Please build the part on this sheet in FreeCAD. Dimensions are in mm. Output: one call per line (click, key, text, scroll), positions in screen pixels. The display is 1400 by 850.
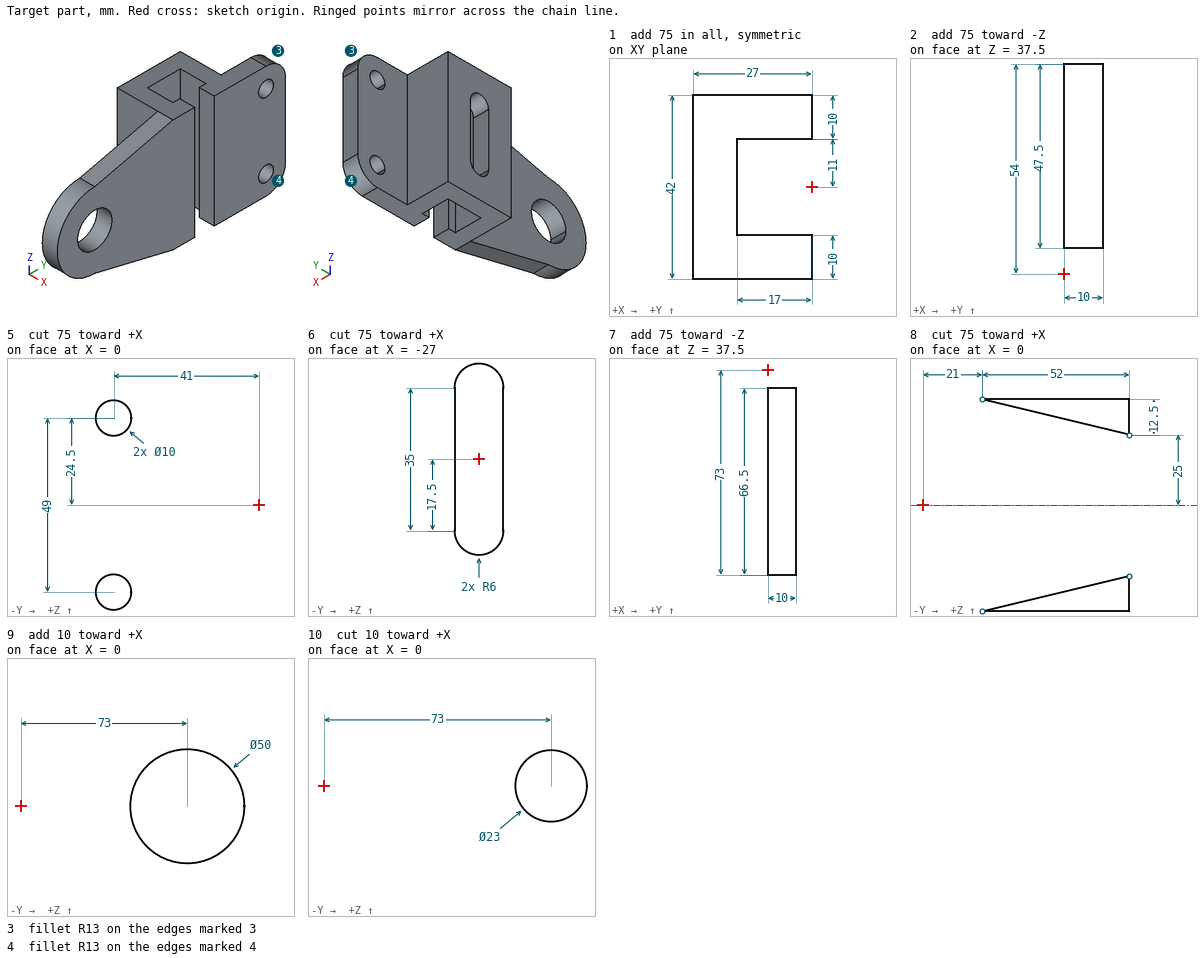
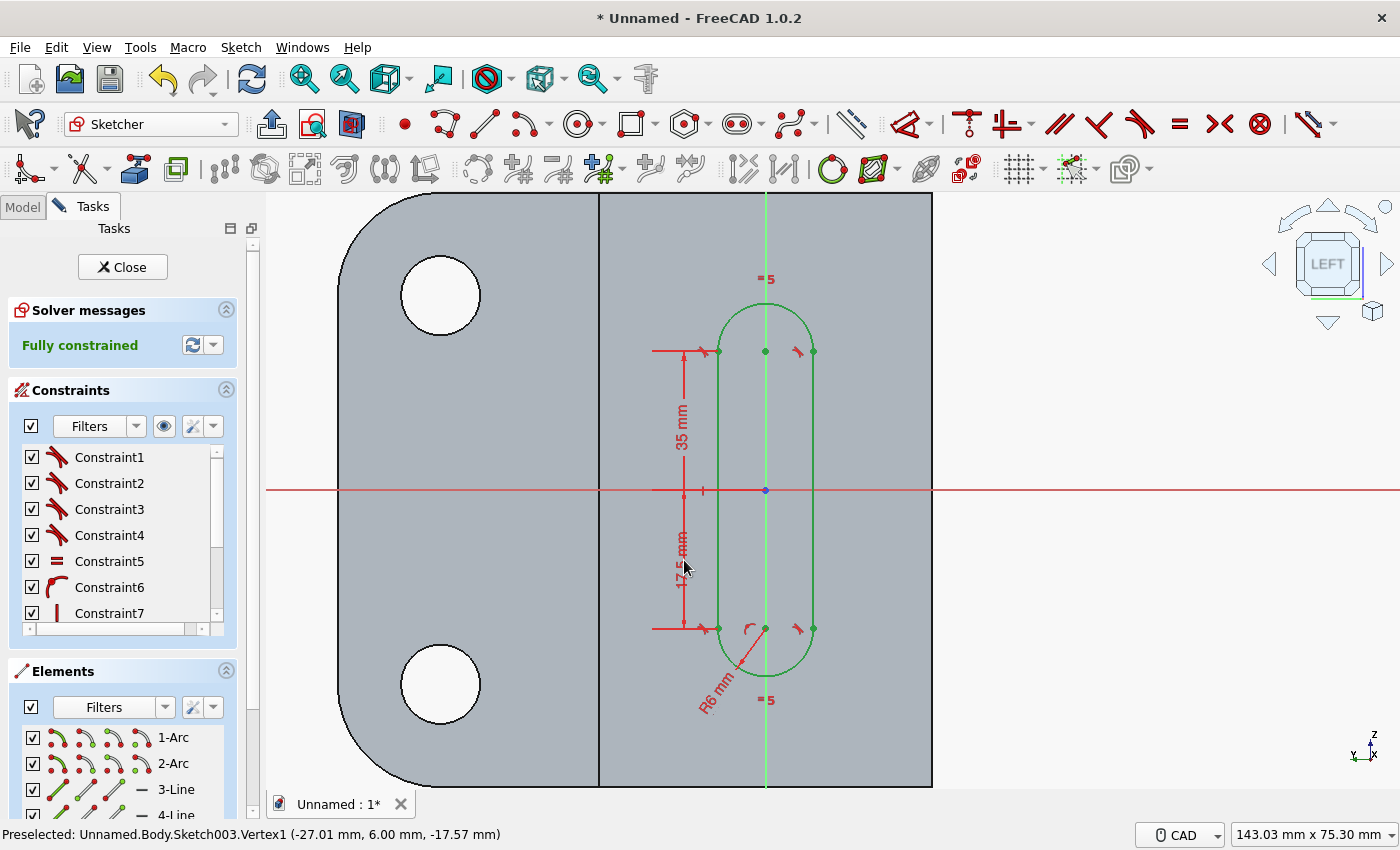
click(123, 267)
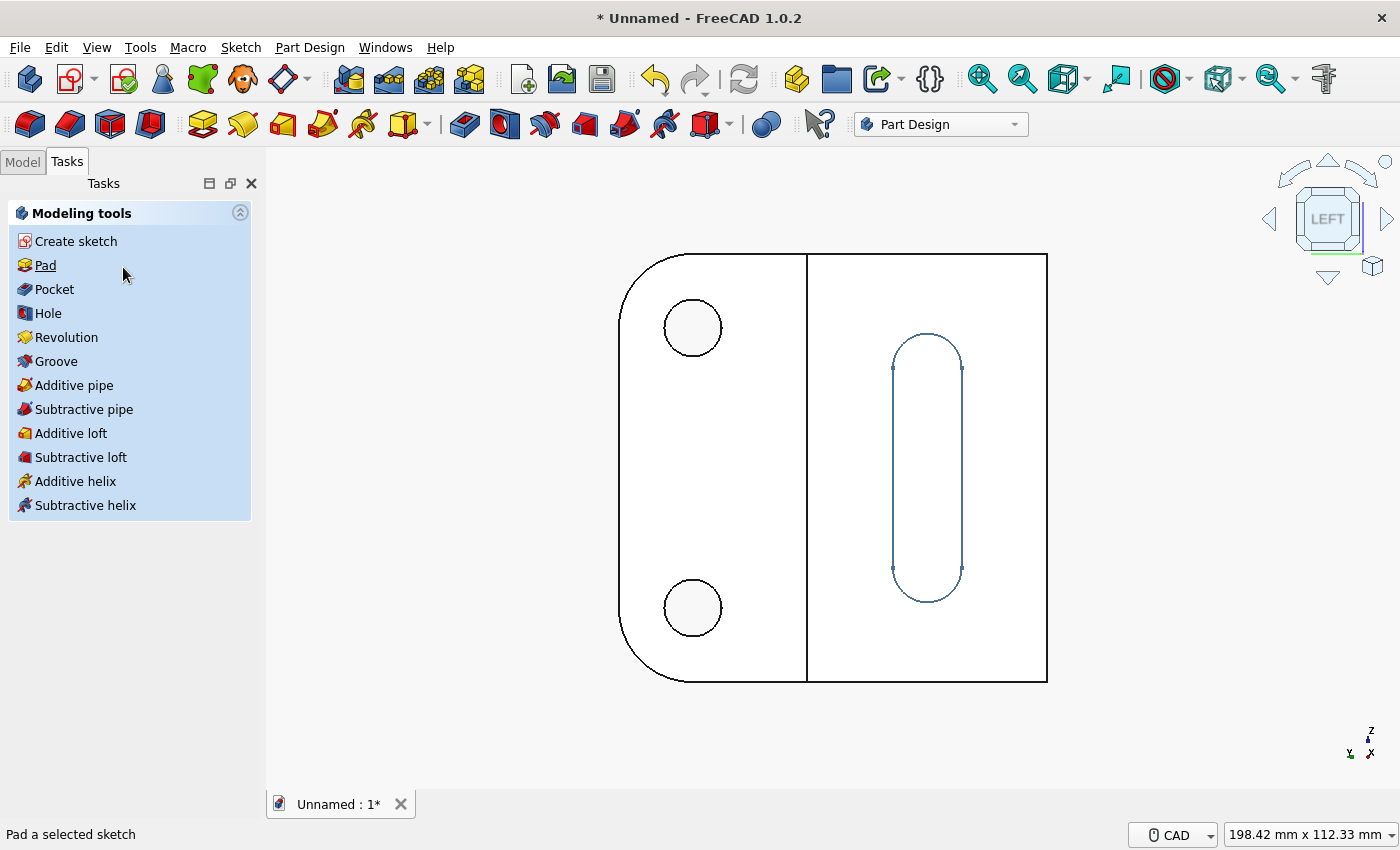
click(466, 124)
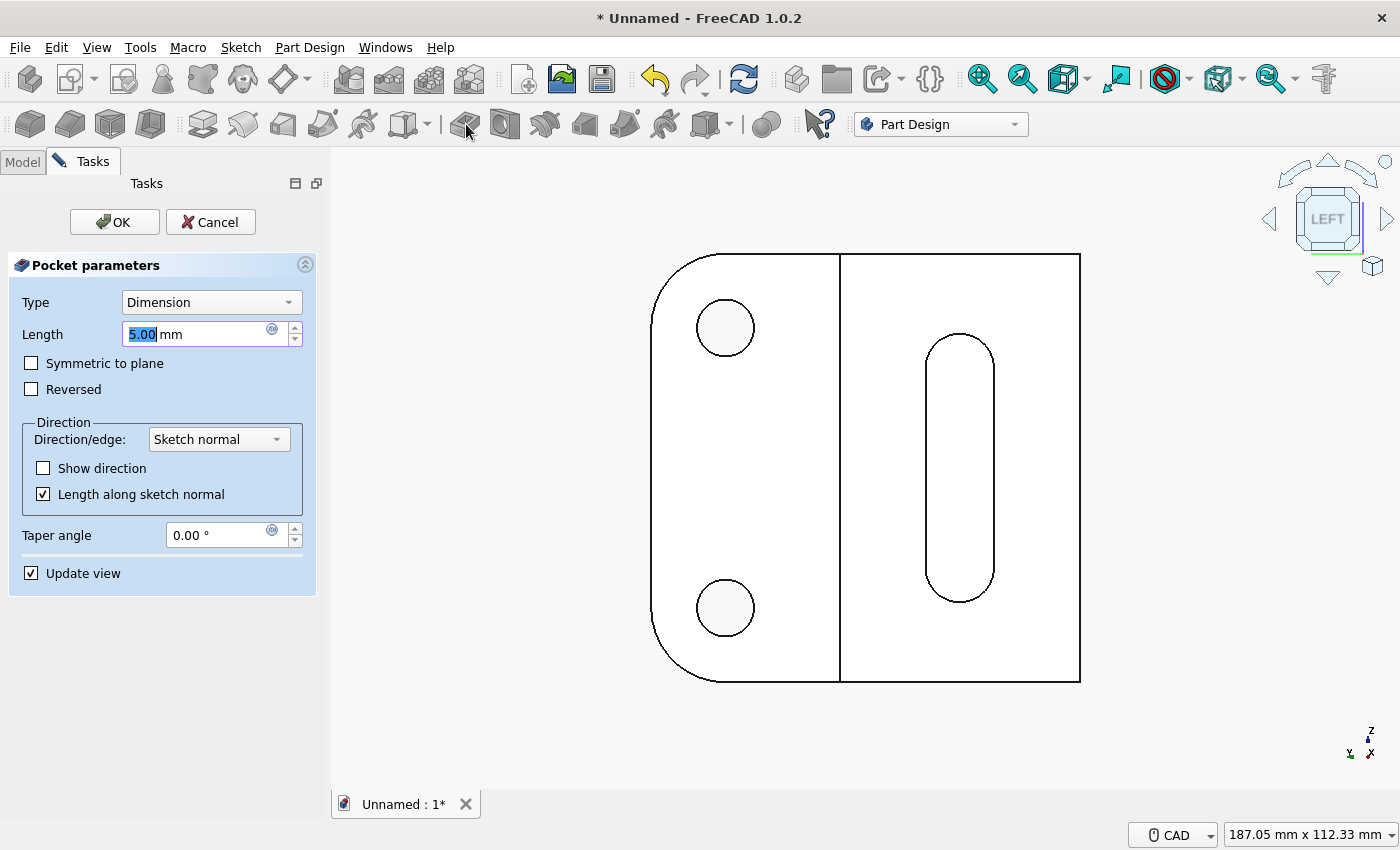
text(75)
key(Tab)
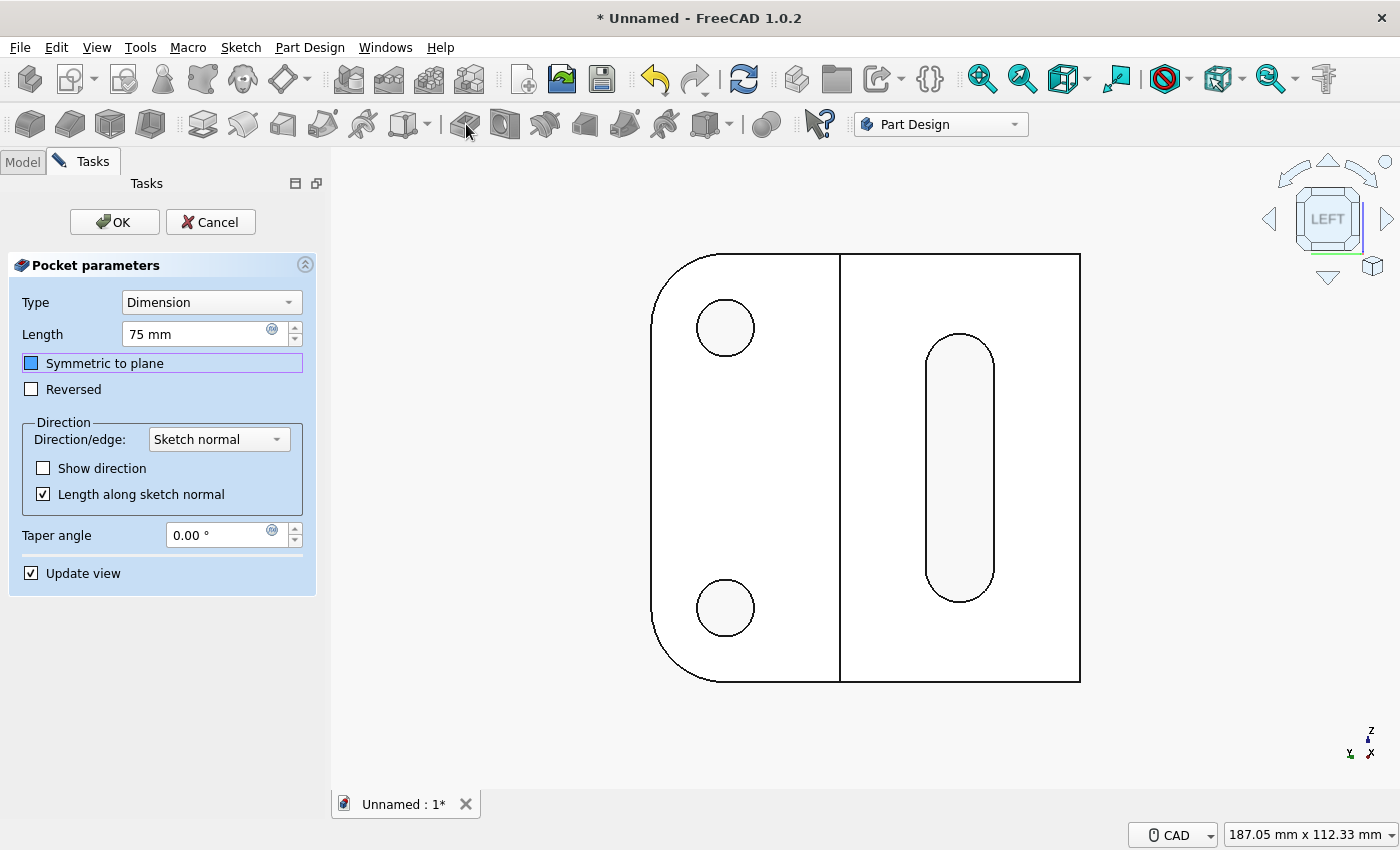
click(115, 222)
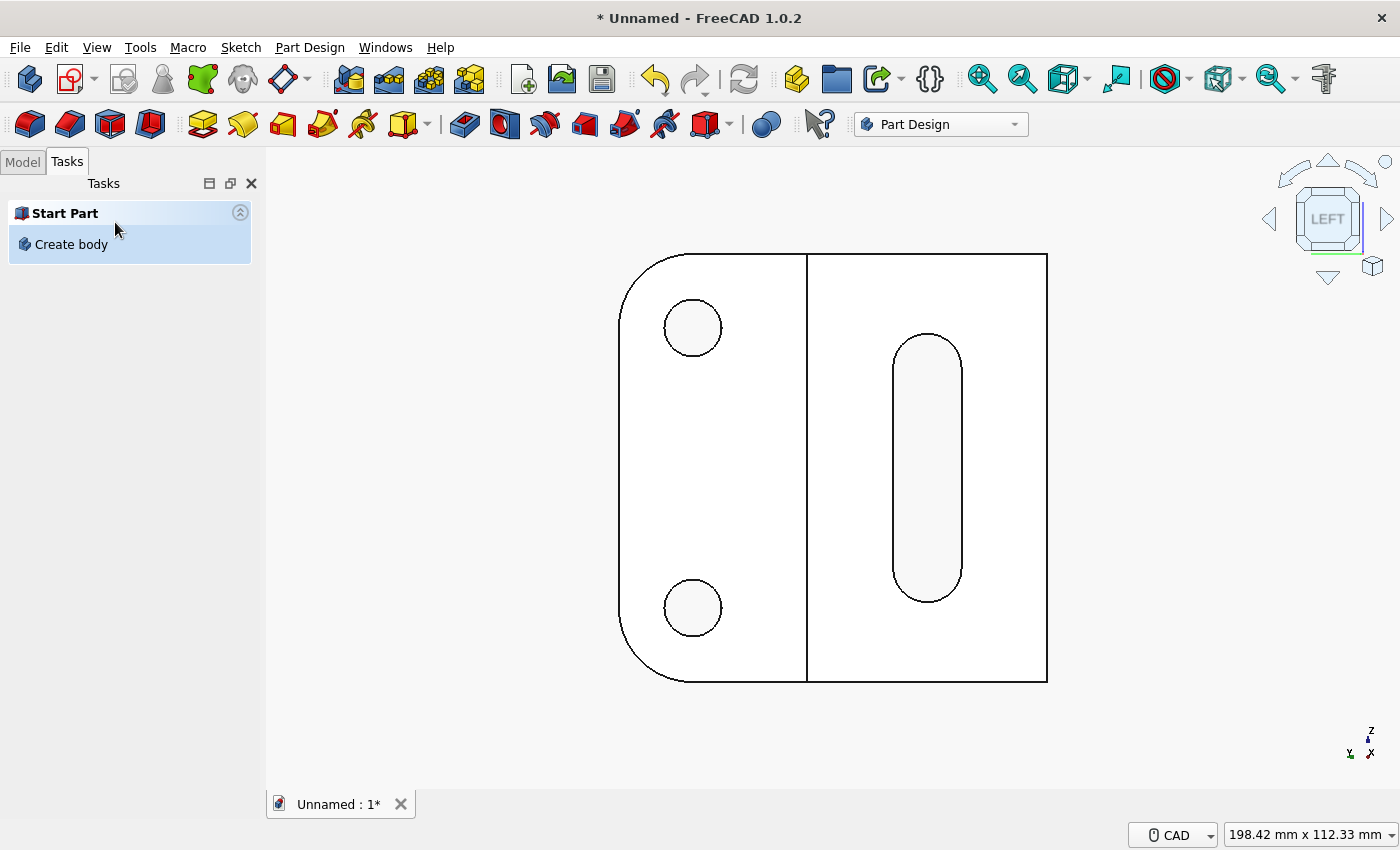
key(0)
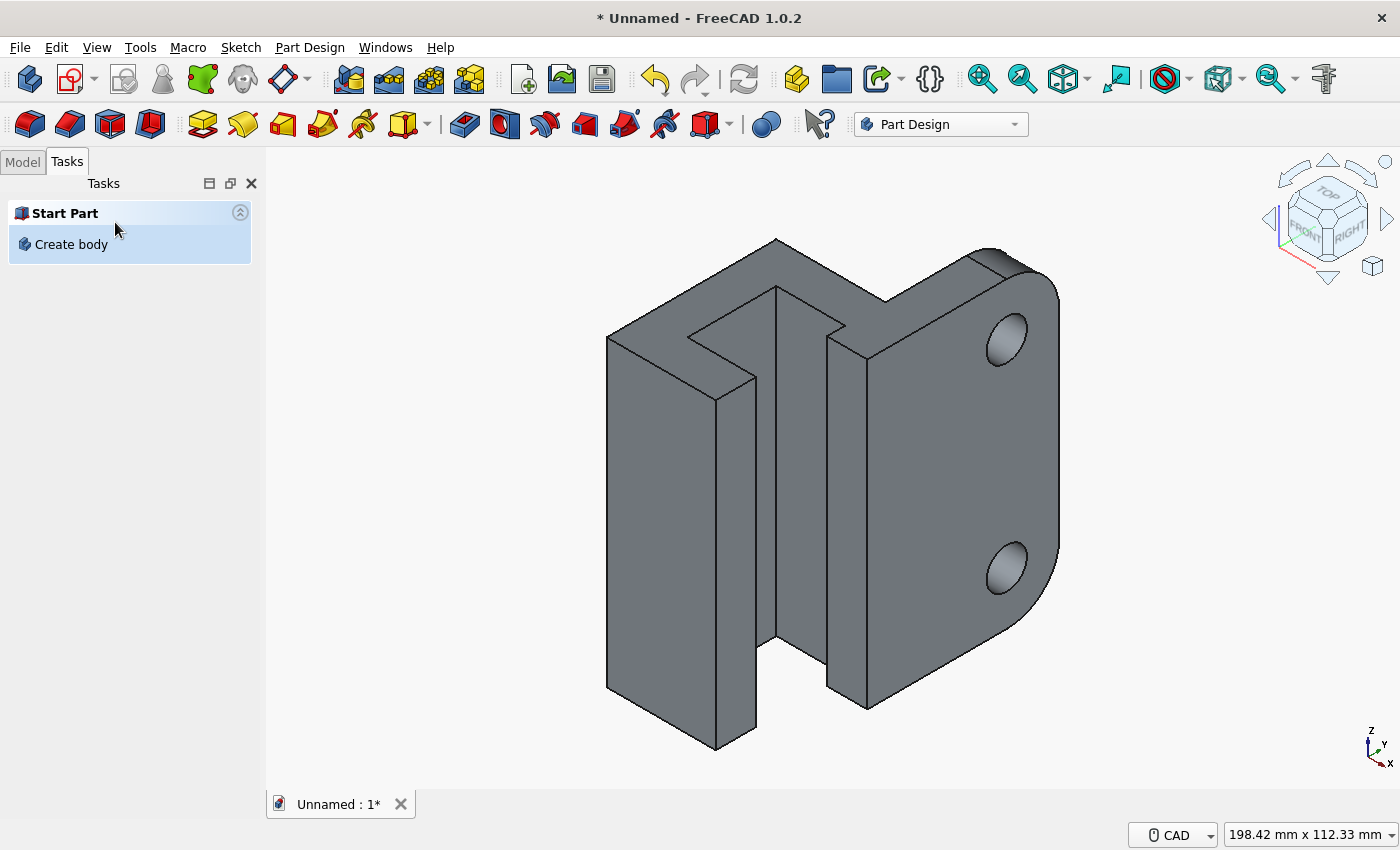
click(699, 369)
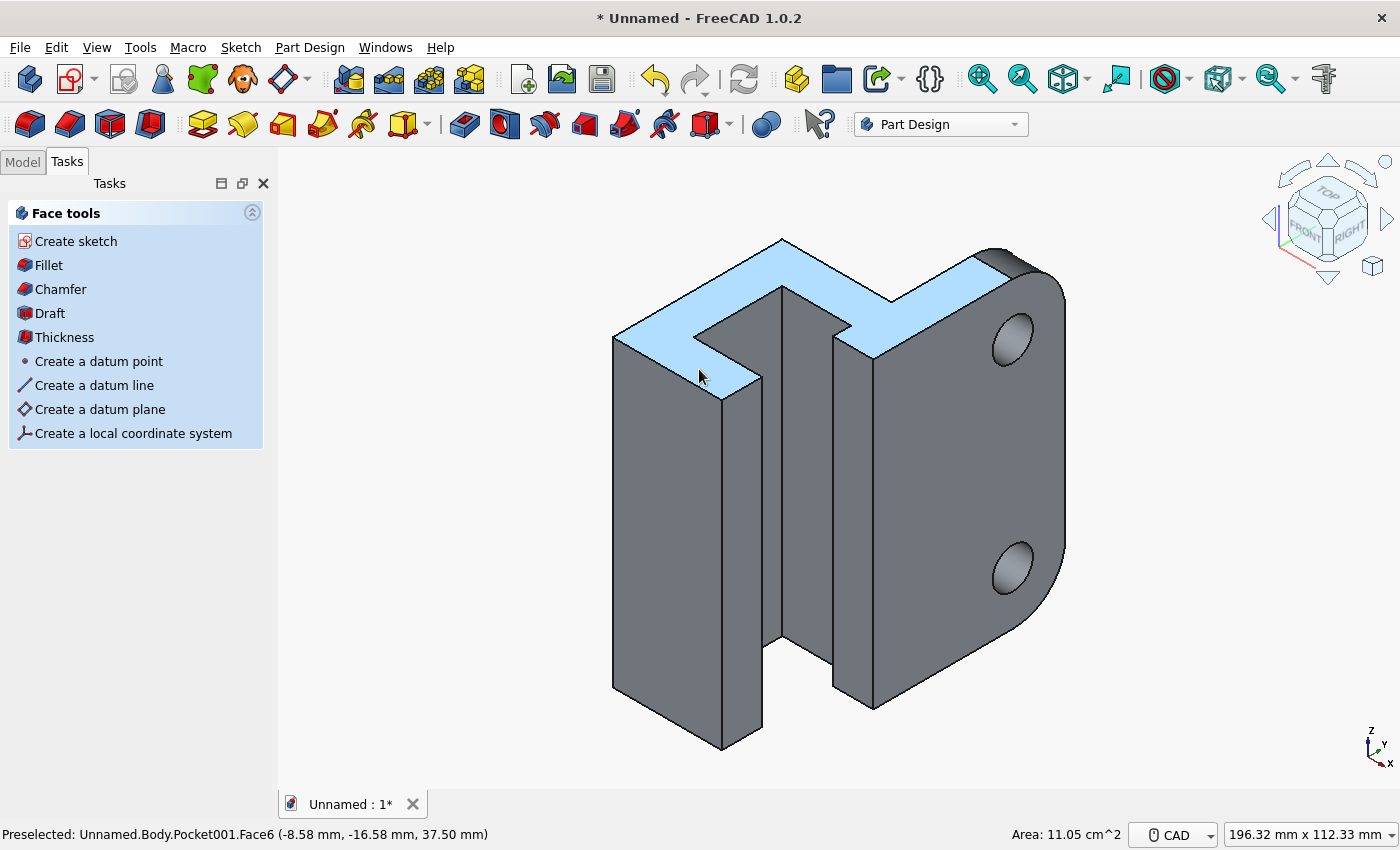
click(70, 80)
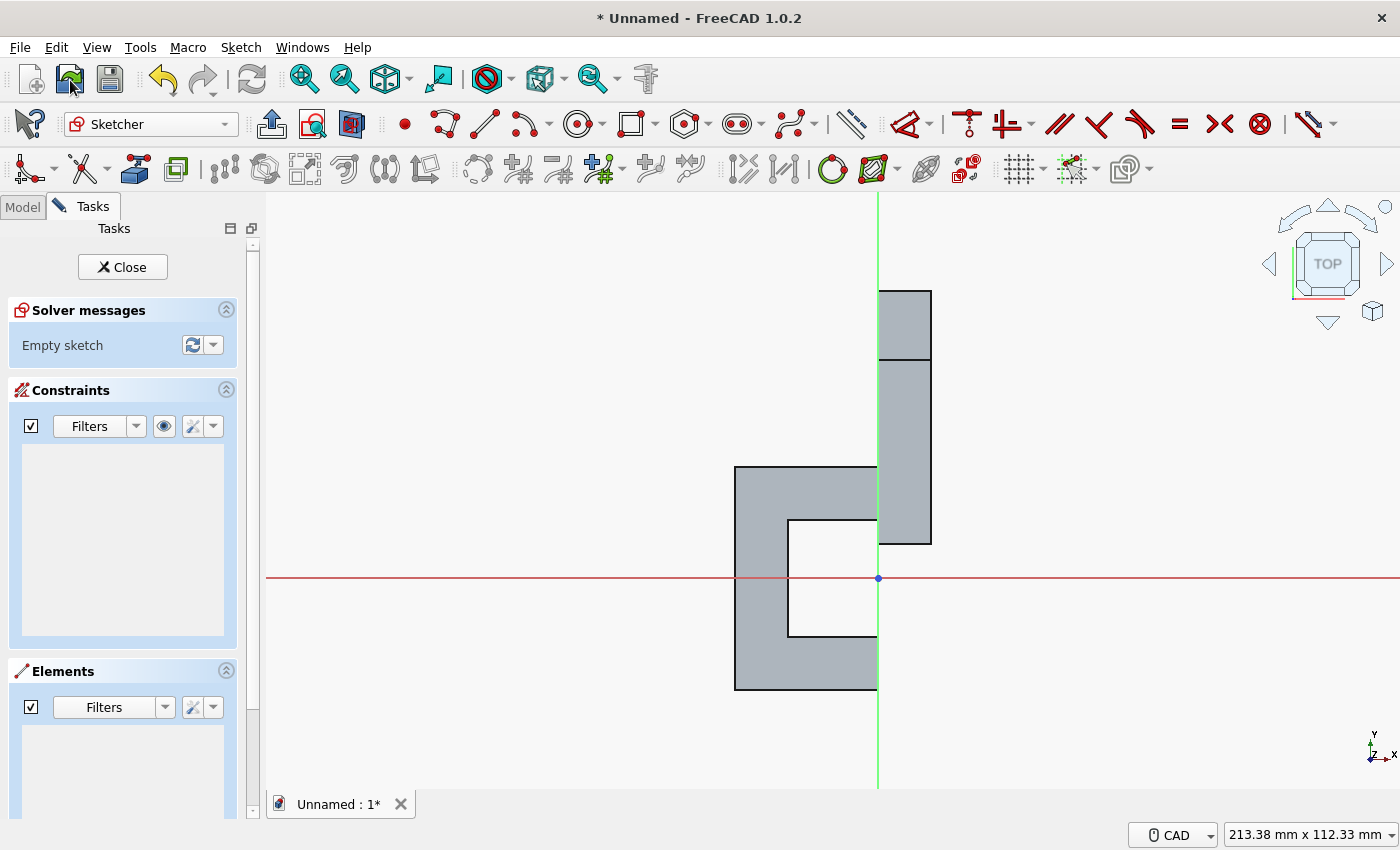
scroll(479, 220, down, 2)